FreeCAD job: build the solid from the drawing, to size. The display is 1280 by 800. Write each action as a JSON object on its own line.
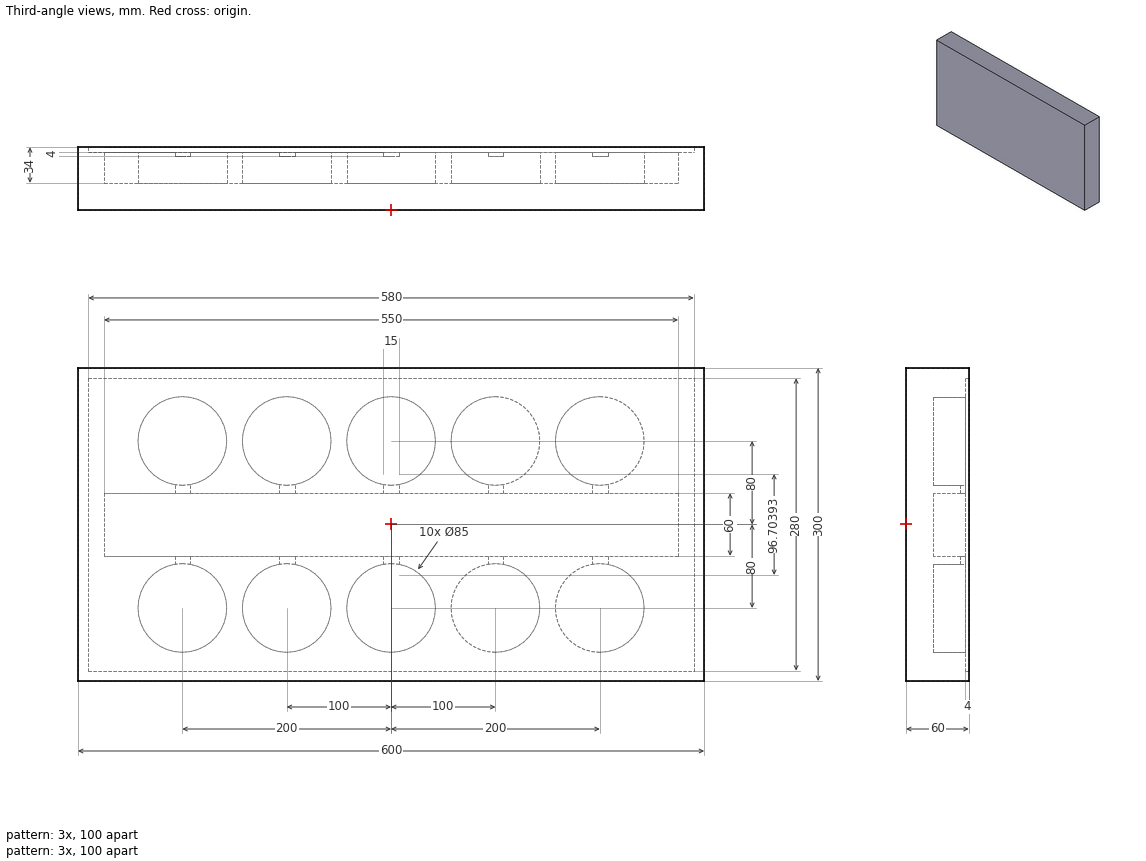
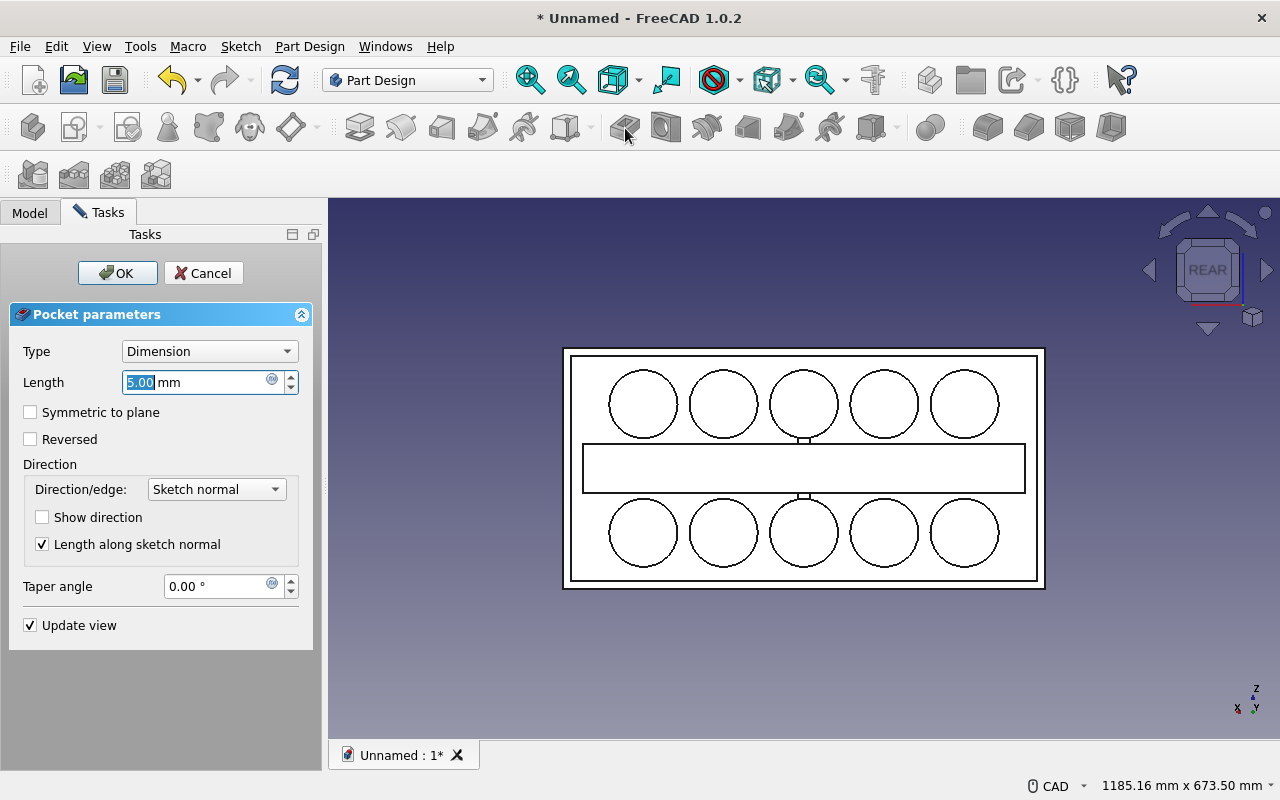
{"action": "type", "text": "4"}
{"action": "key", "text": "Tab"}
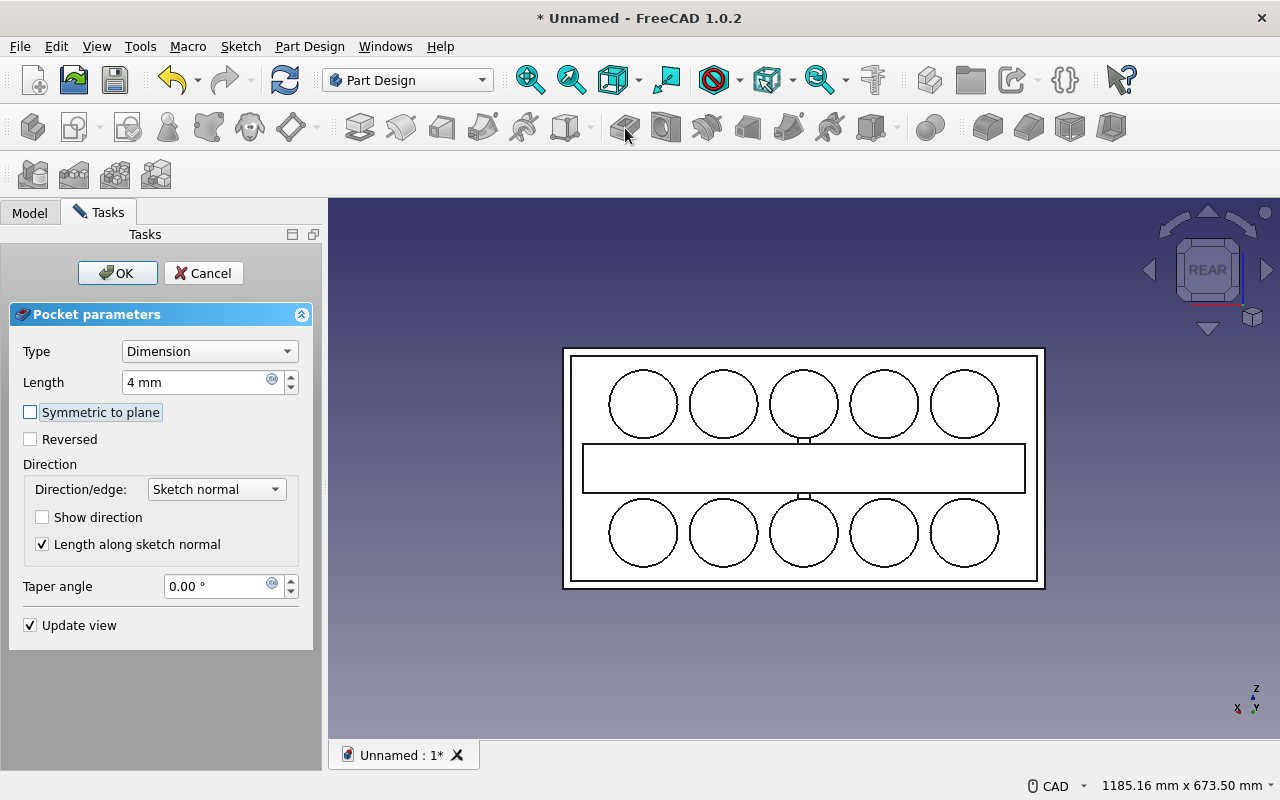
{"action": "left_click", "coordinate": [118, 273]}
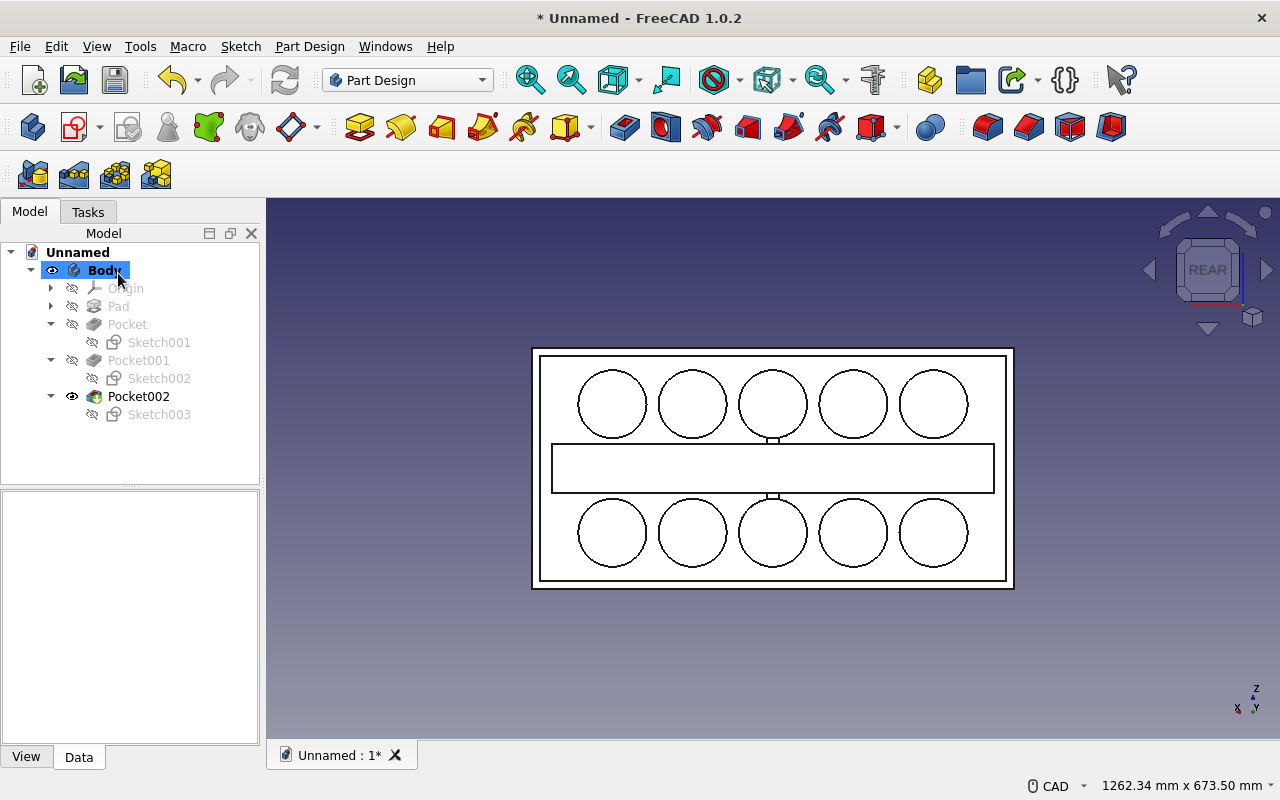
{"action": "left_click", "coordinate": [117, 396]}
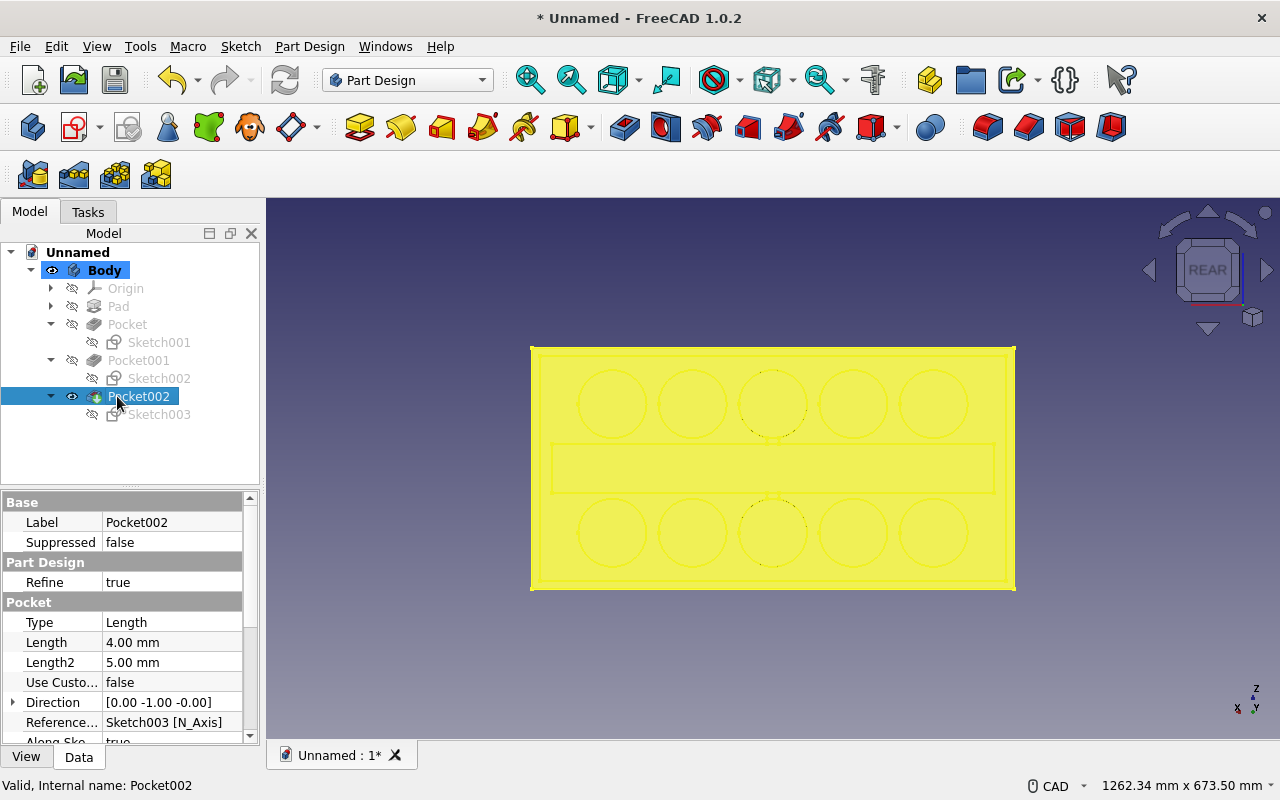
{"action": "left_click", "coordinate": [74, 174]}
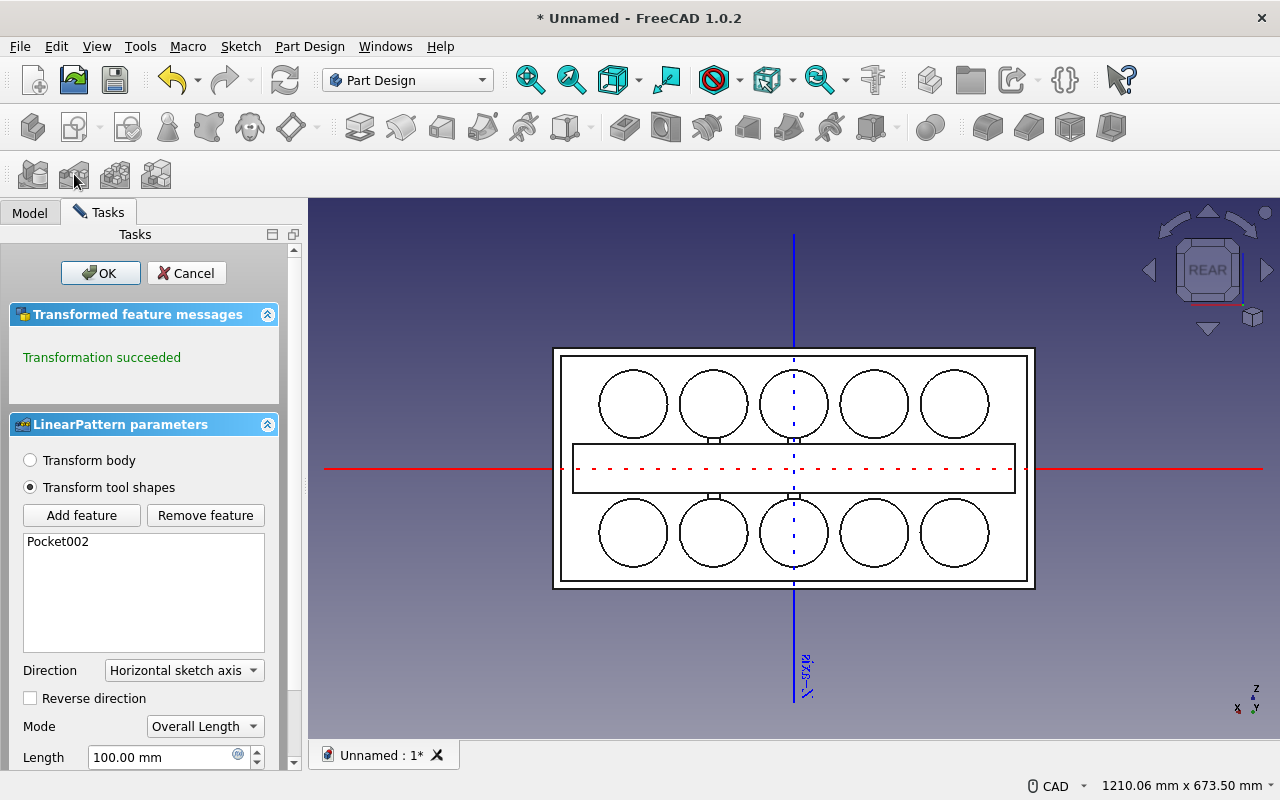
{"action": "left_click", "coordinate": [185, 670]}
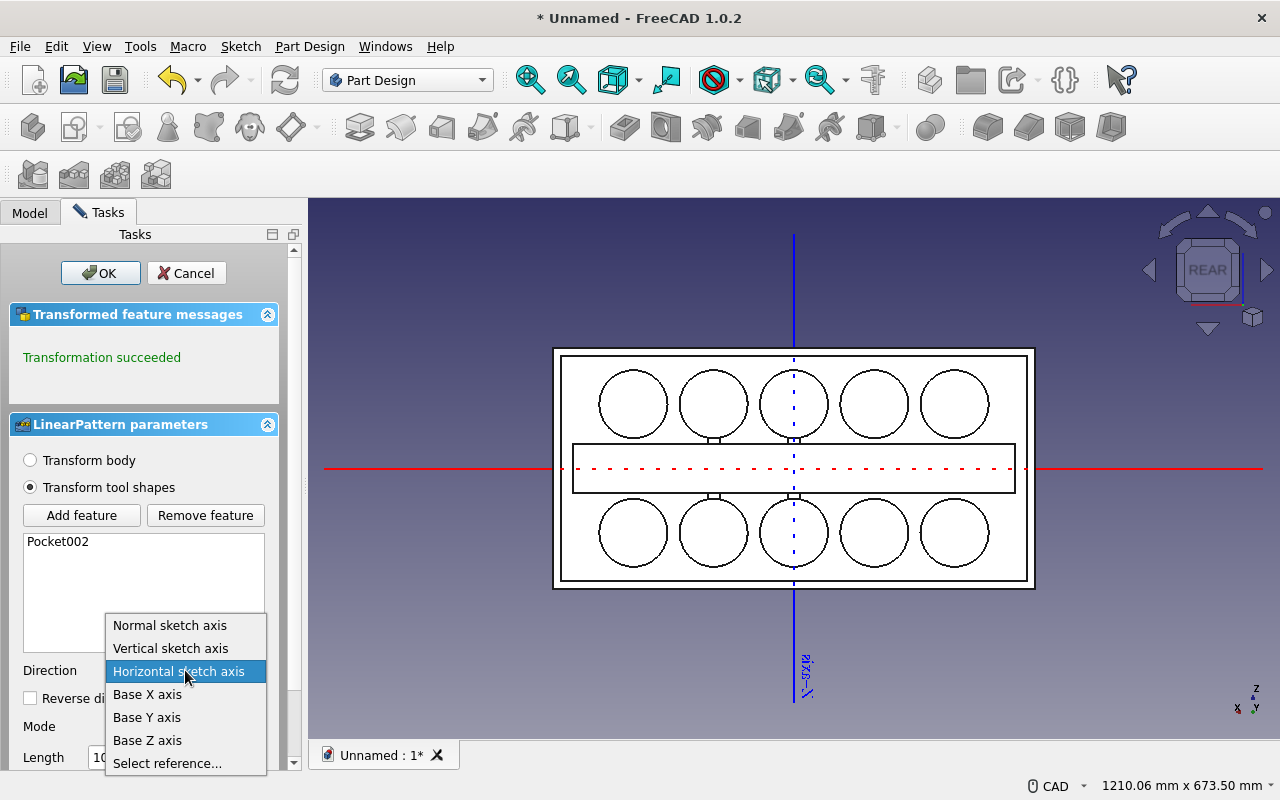
{"action": "left_click", "coordinate": [184, 694]}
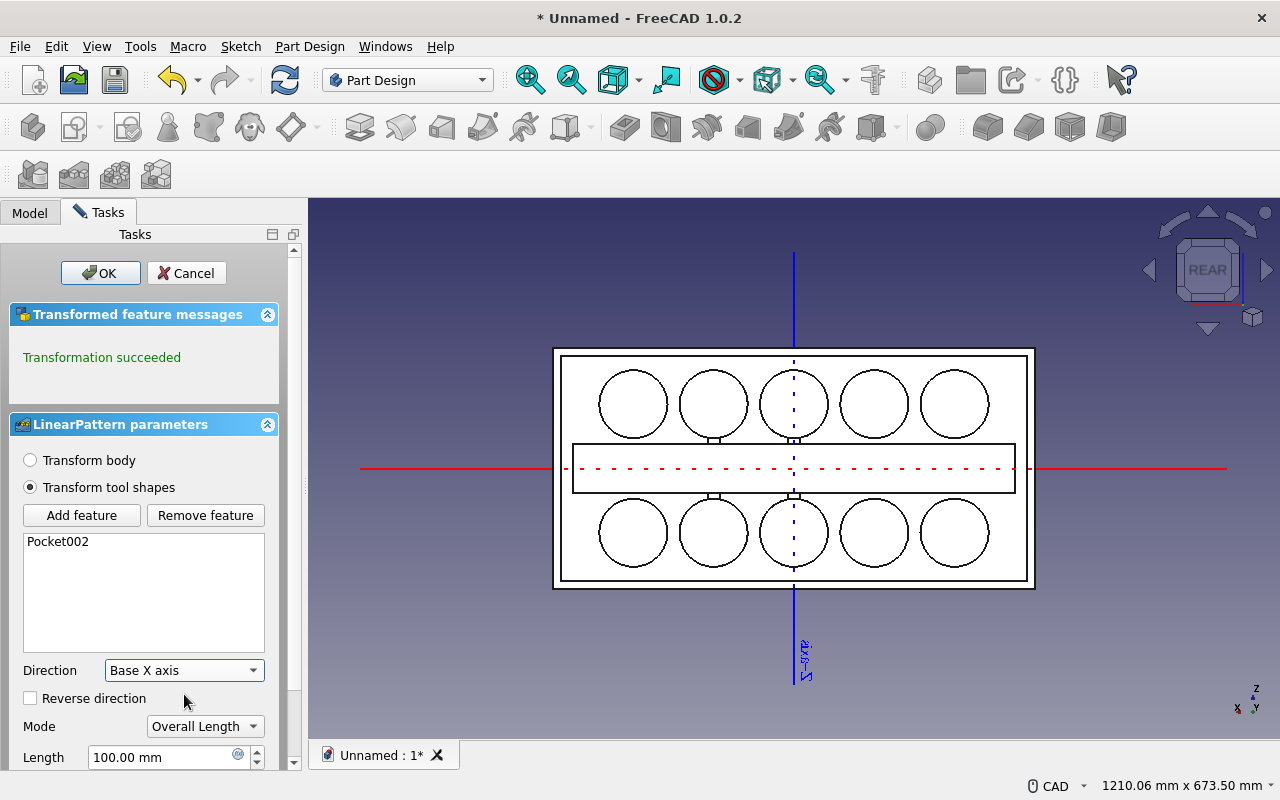
{"action": "left_click", "coordinate": [206, 726]}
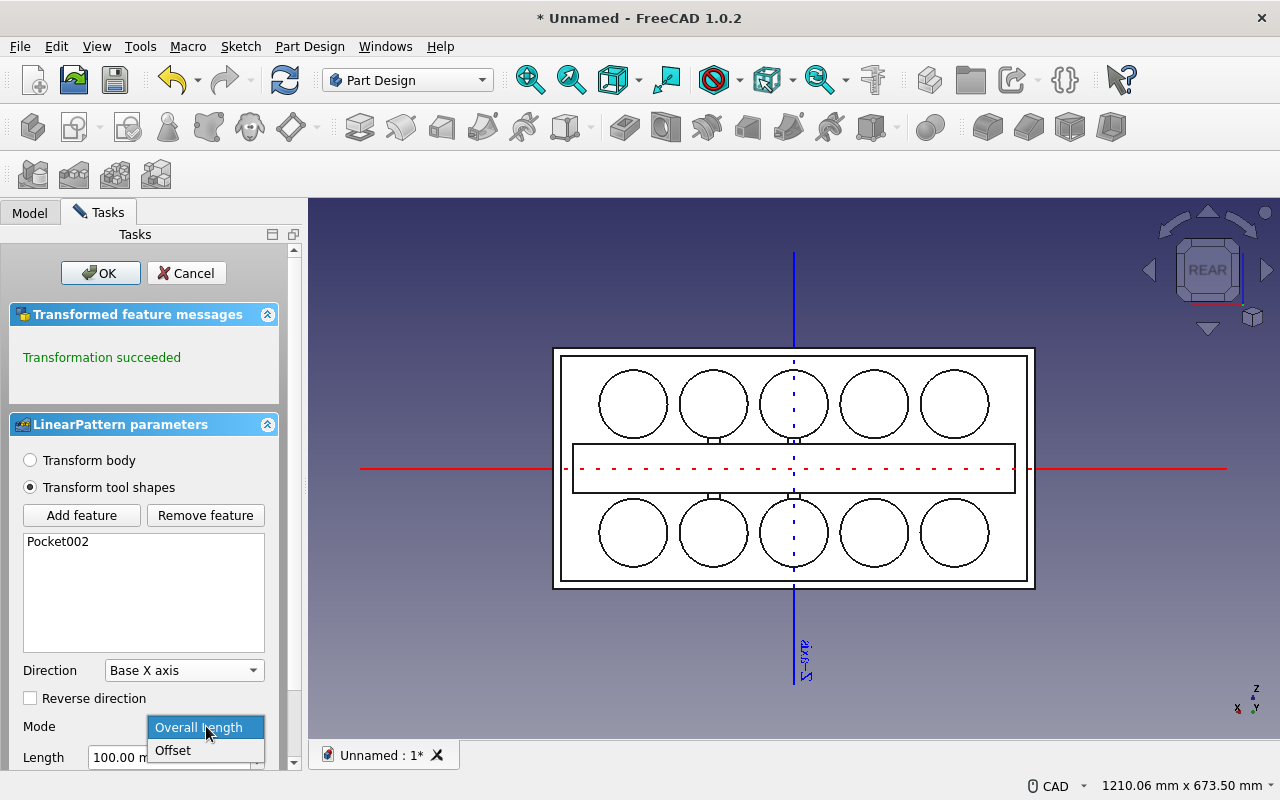
{"action": "left_click", "coordinate": [204, 750]}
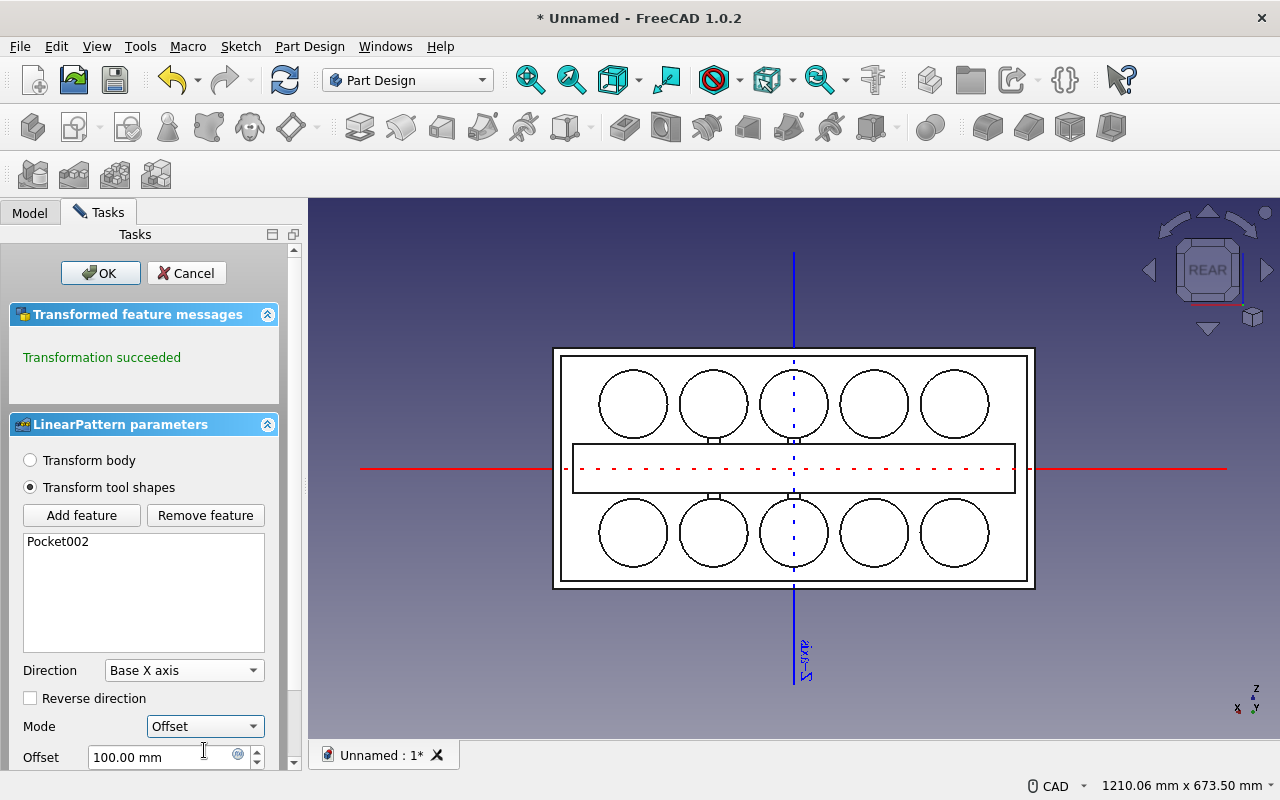
{"action": "scroll", "coordinate": [294, 507], "scroll_direction": "down", "scroll_amount": 2}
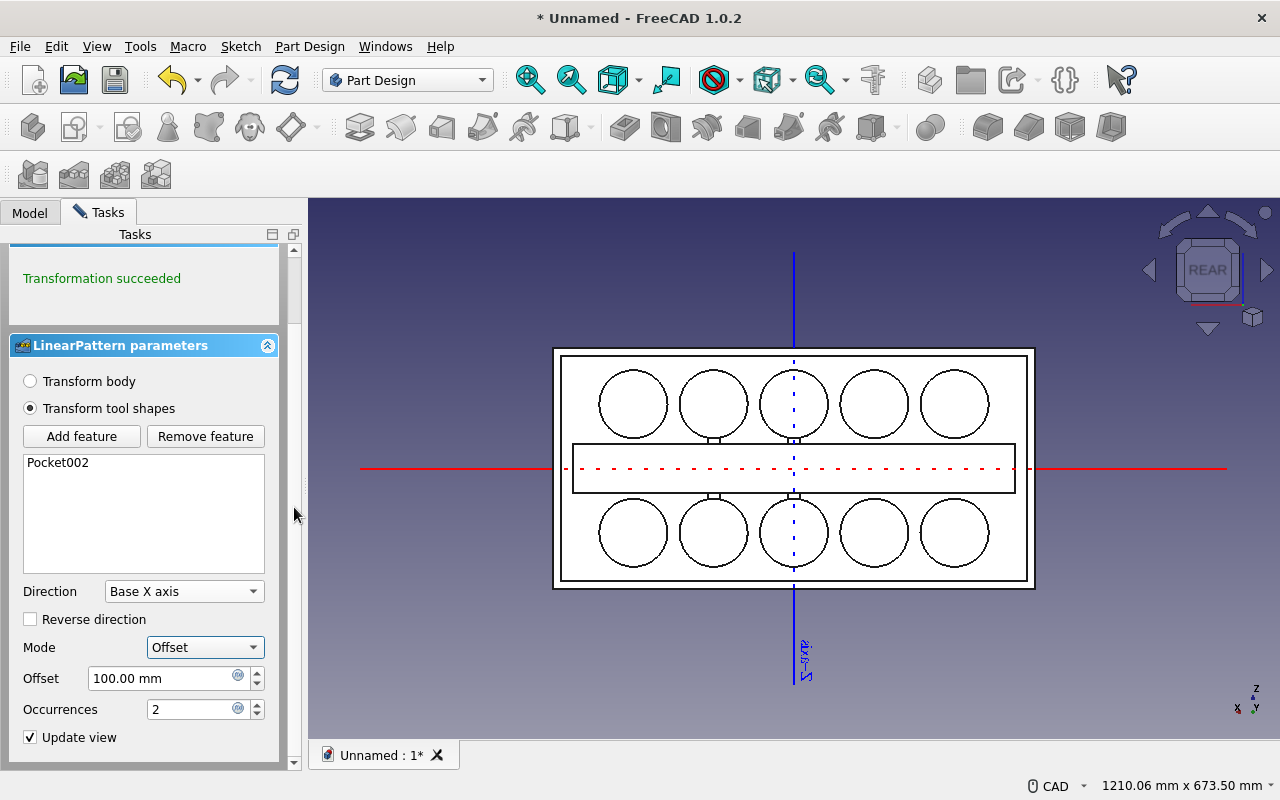
{"action": "triple_click", "coordinate": [170, 678]}